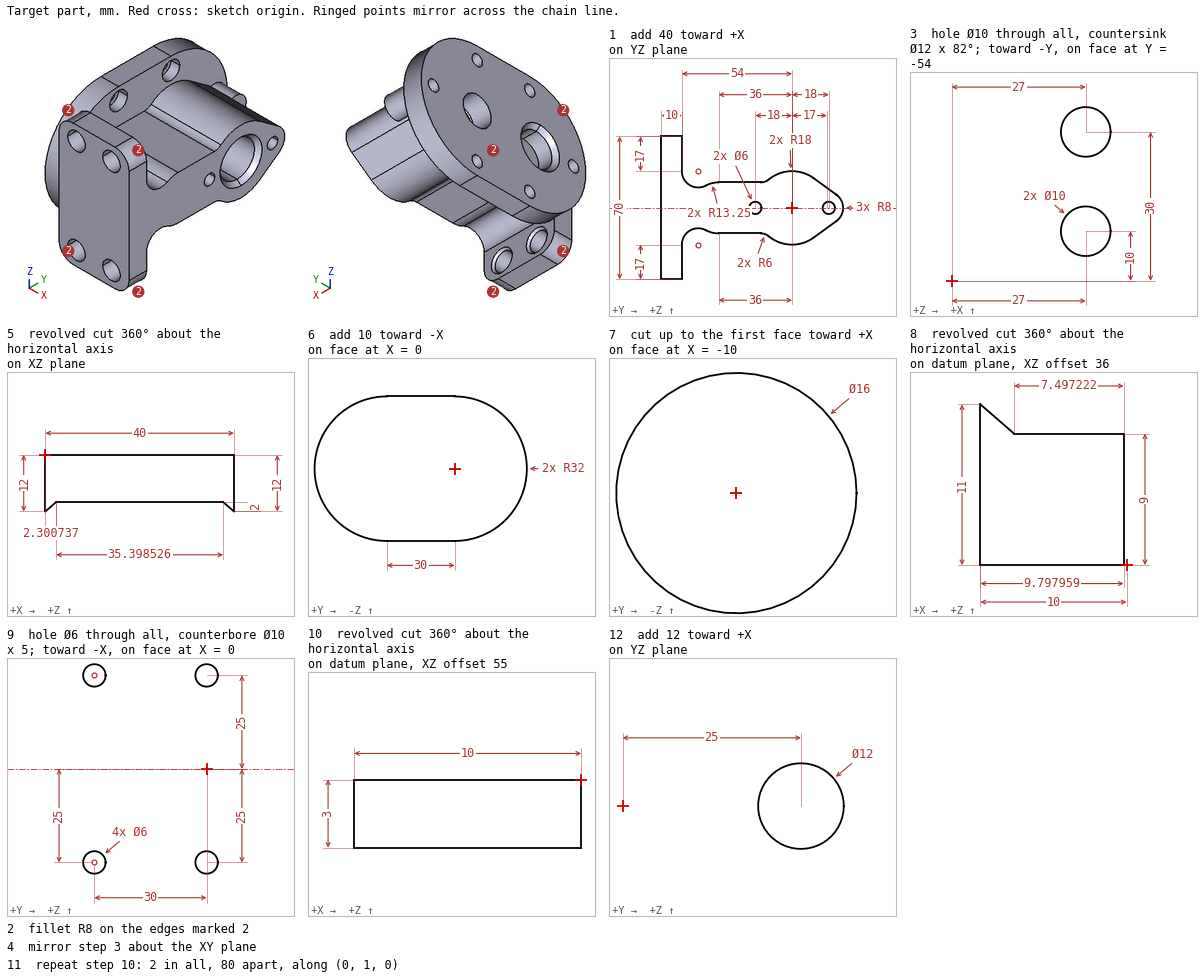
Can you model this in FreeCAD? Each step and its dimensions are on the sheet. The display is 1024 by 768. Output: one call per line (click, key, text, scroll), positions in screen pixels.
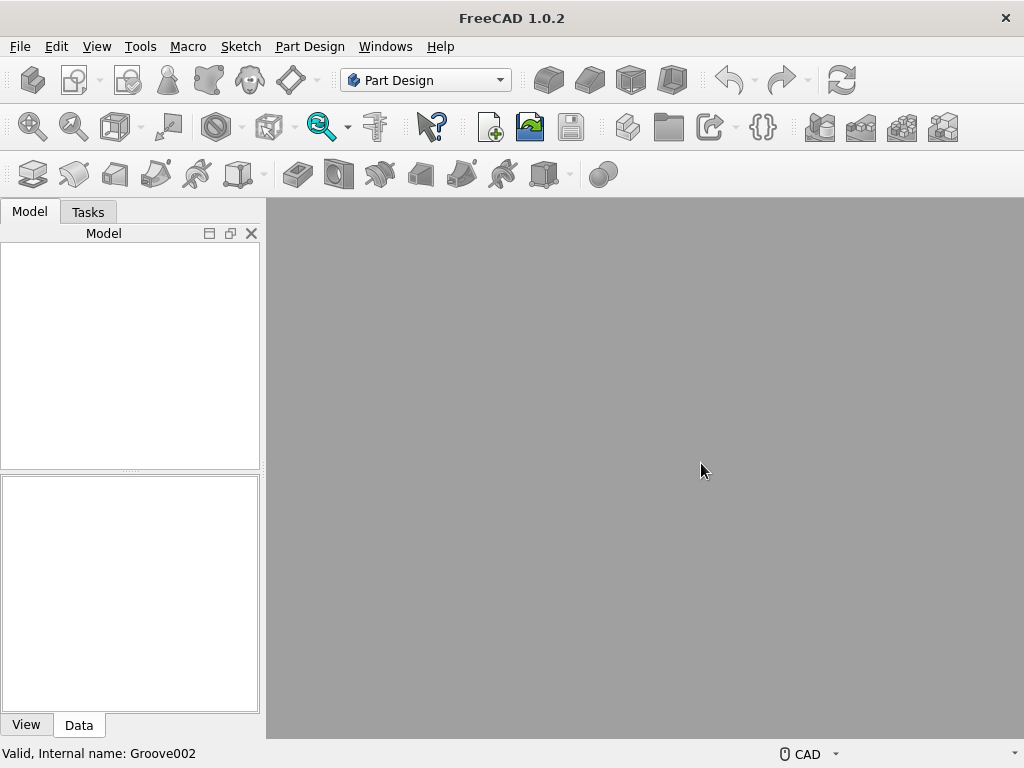
click(489, 128)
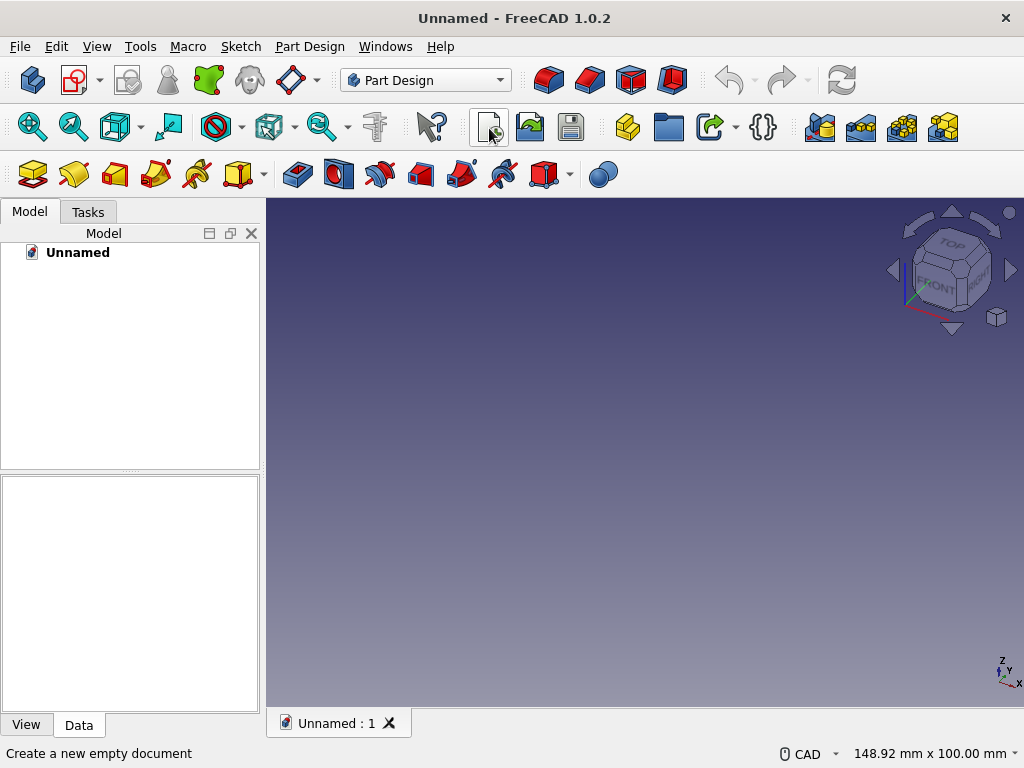
click(74, 80)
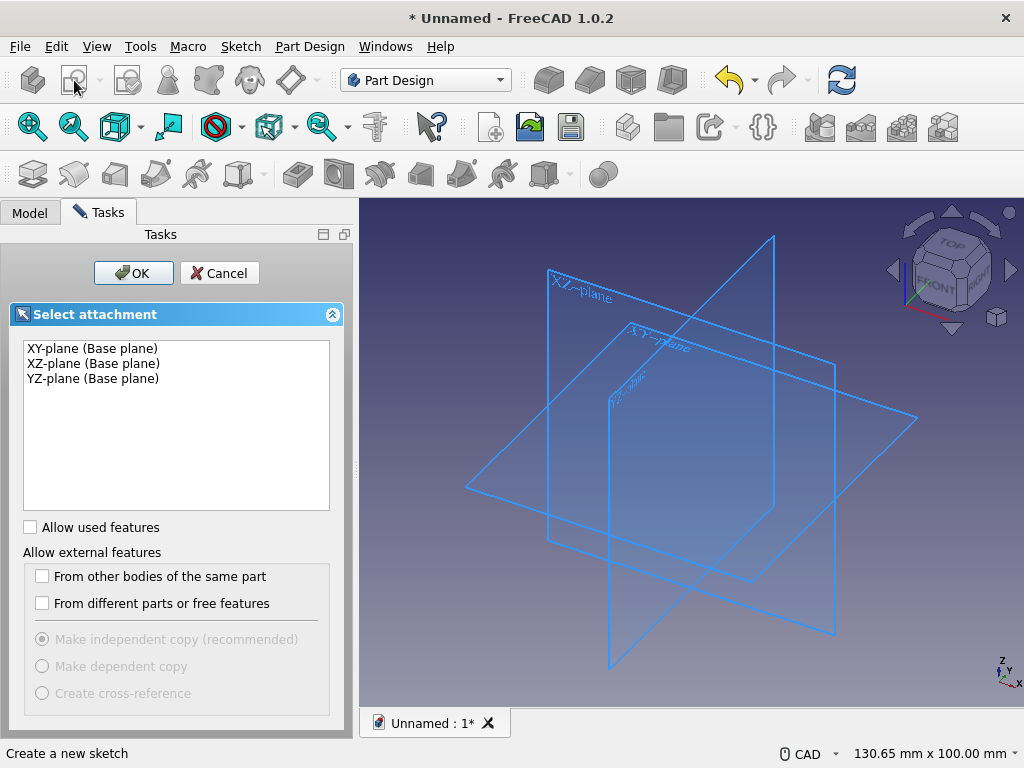
click(84, 378)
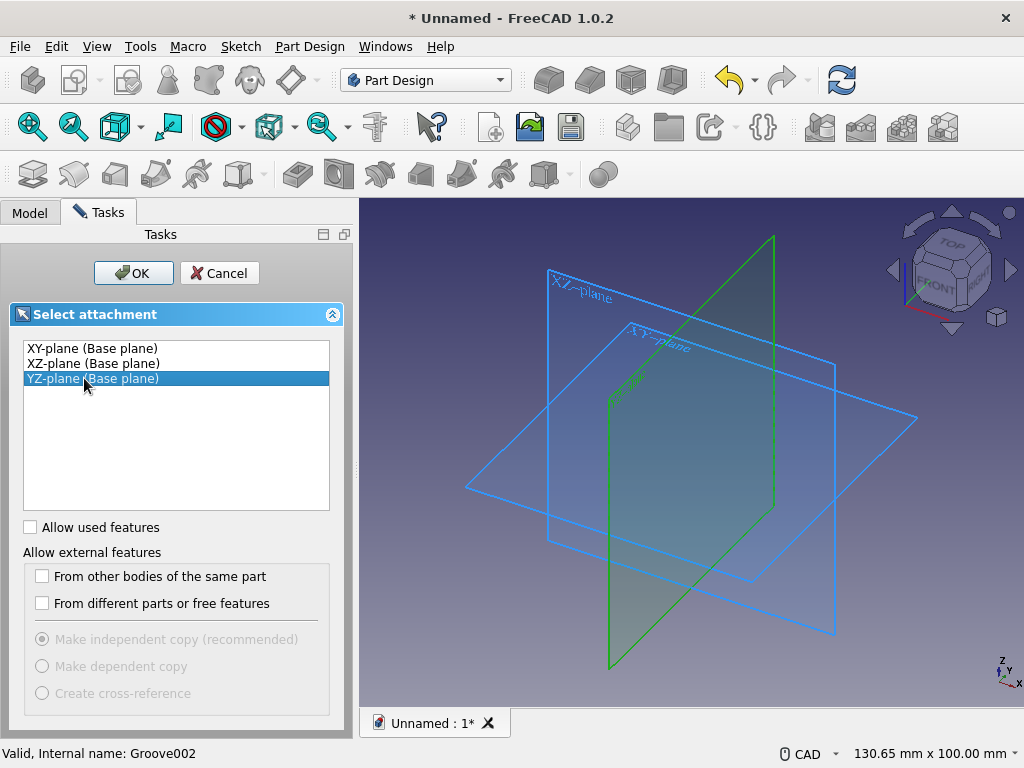
click(134, 273)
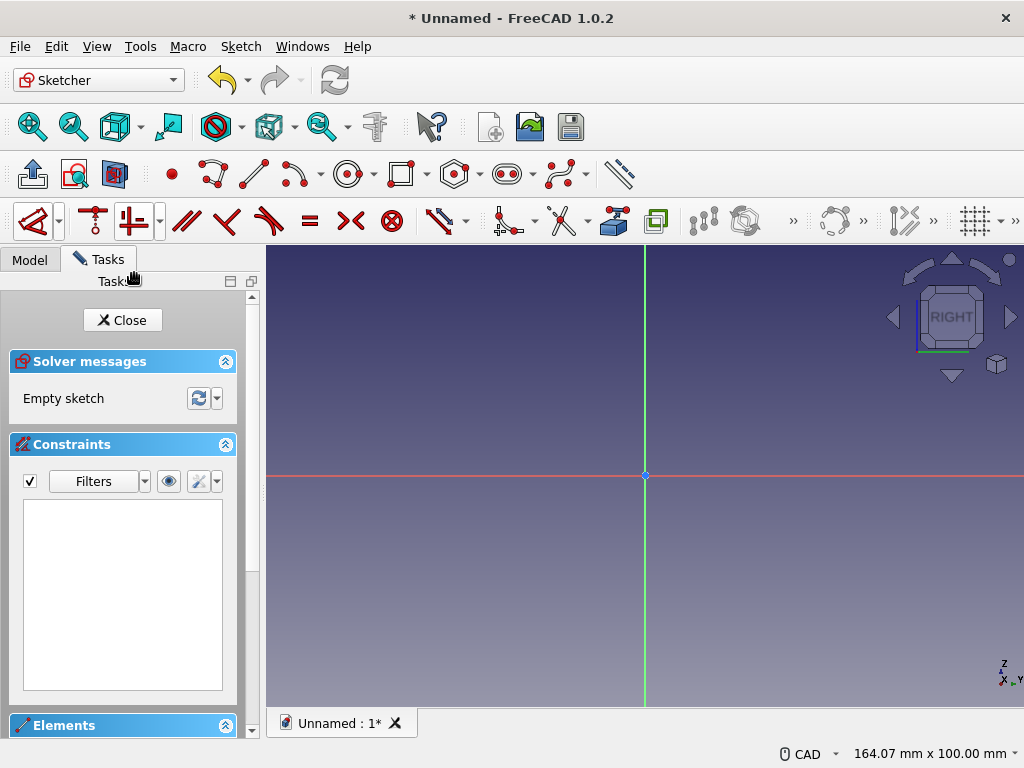
click(254, 174)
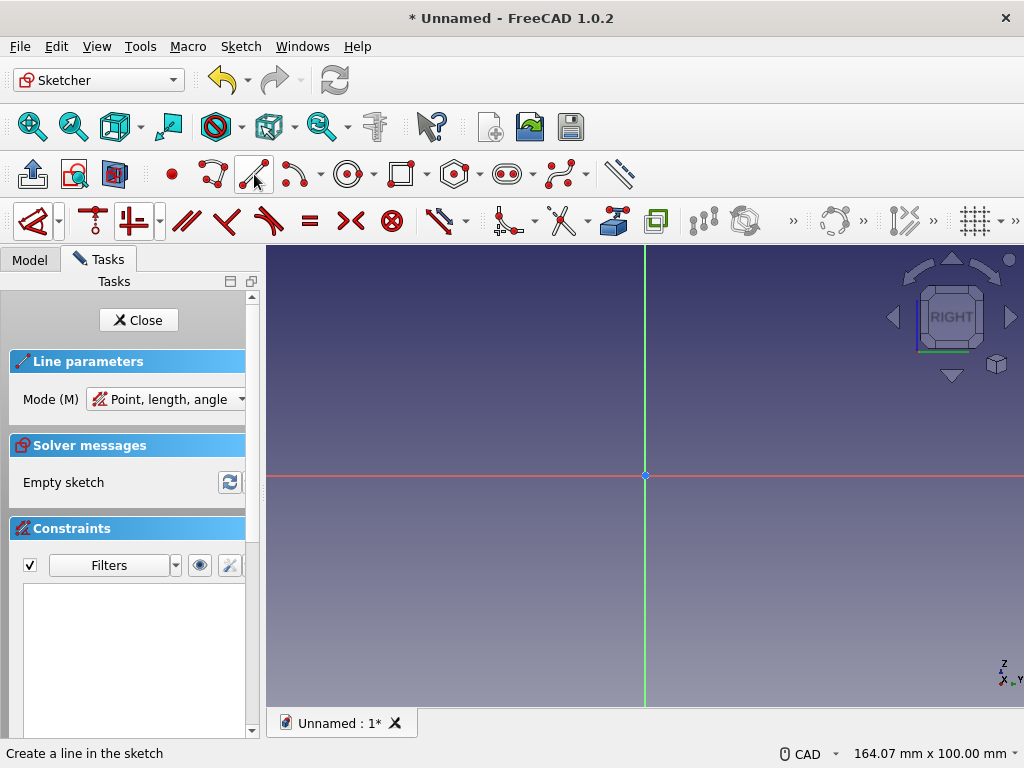
click(574, 418)
click(479, 418)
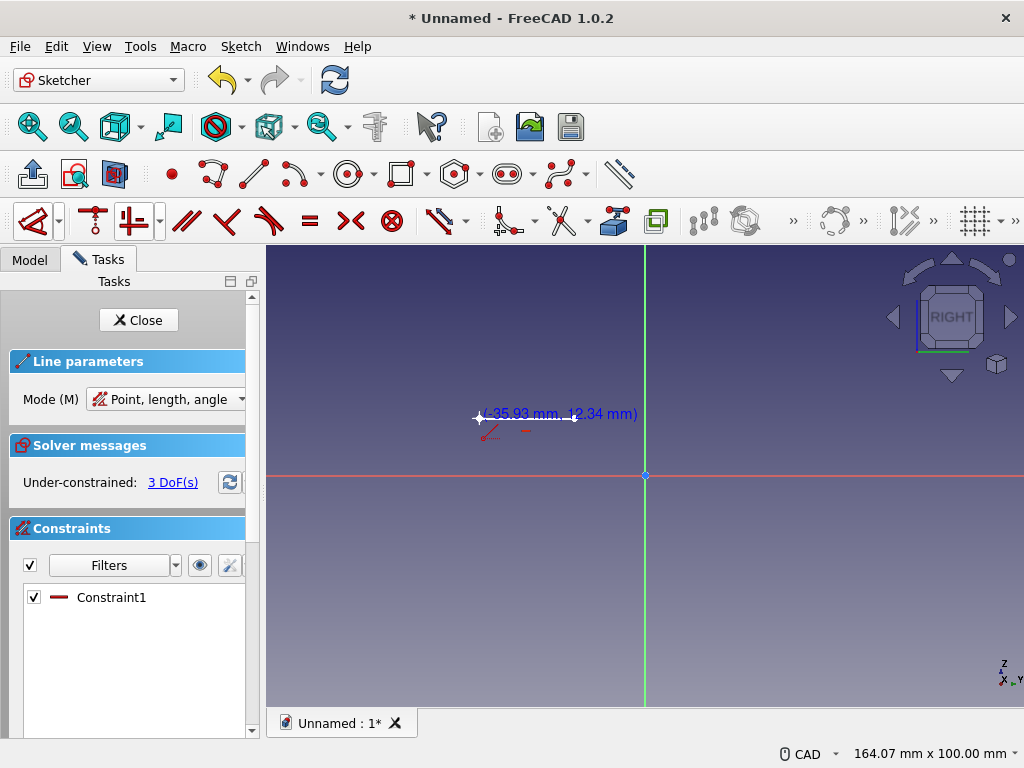
click(213, 174)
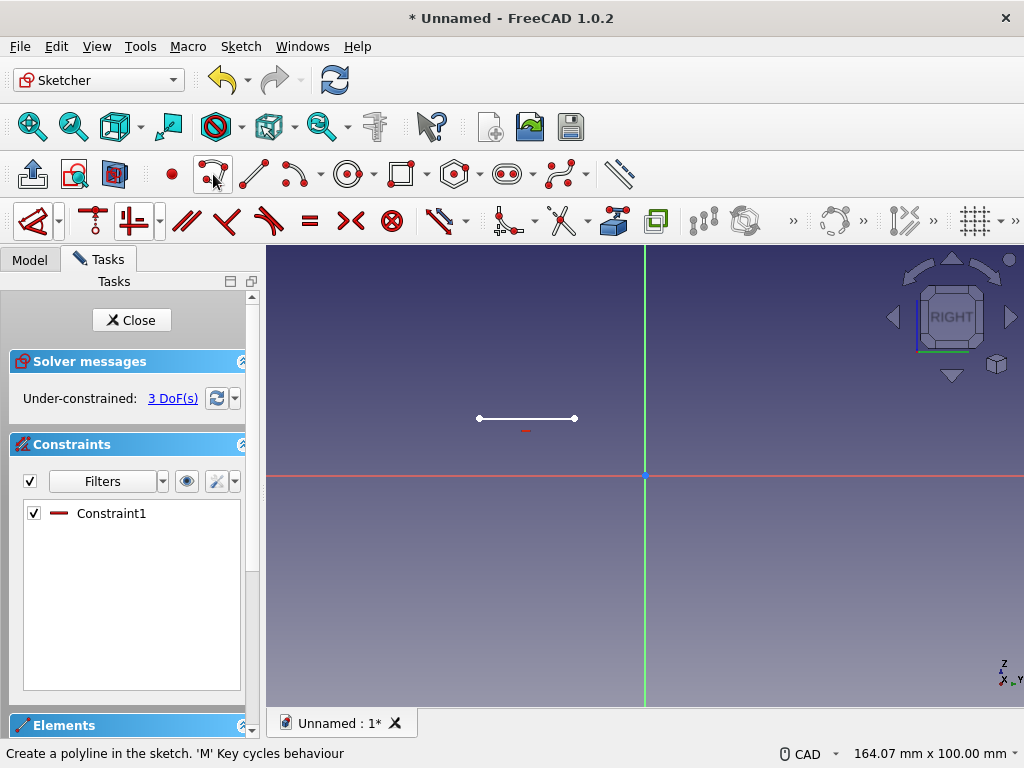
click(396, 393)
click(396, 314)
click(349, 314)
click(349, 638)
click(396, 638)
click(396, 559)
right_click(396, 559)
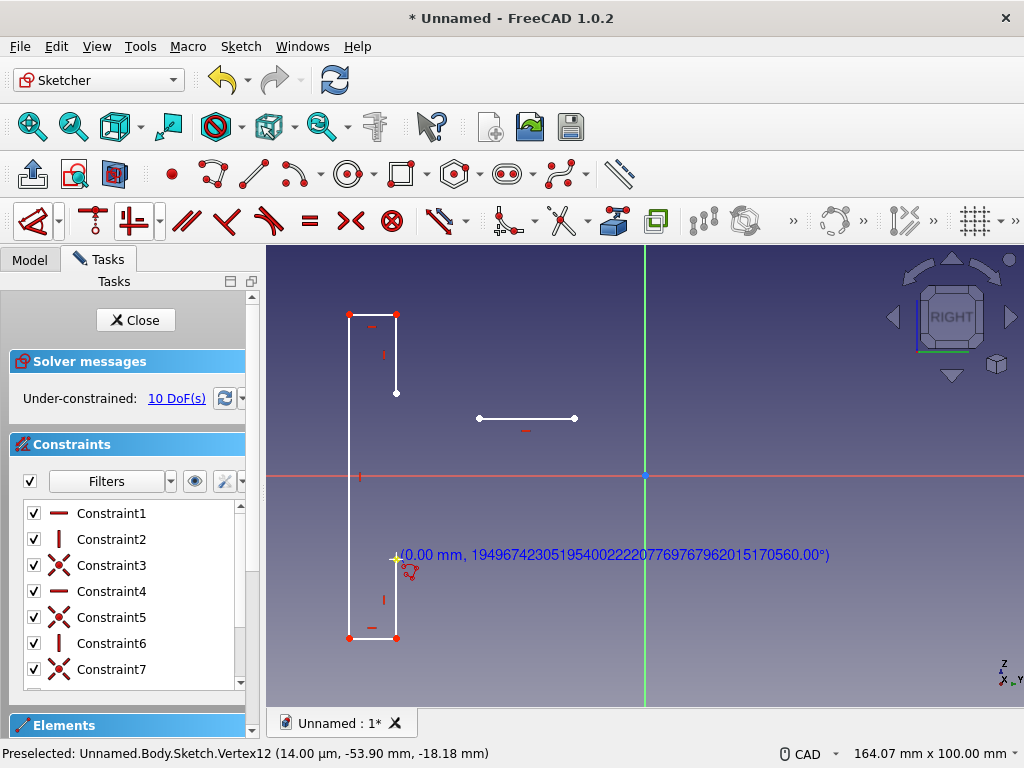
click(254, 174)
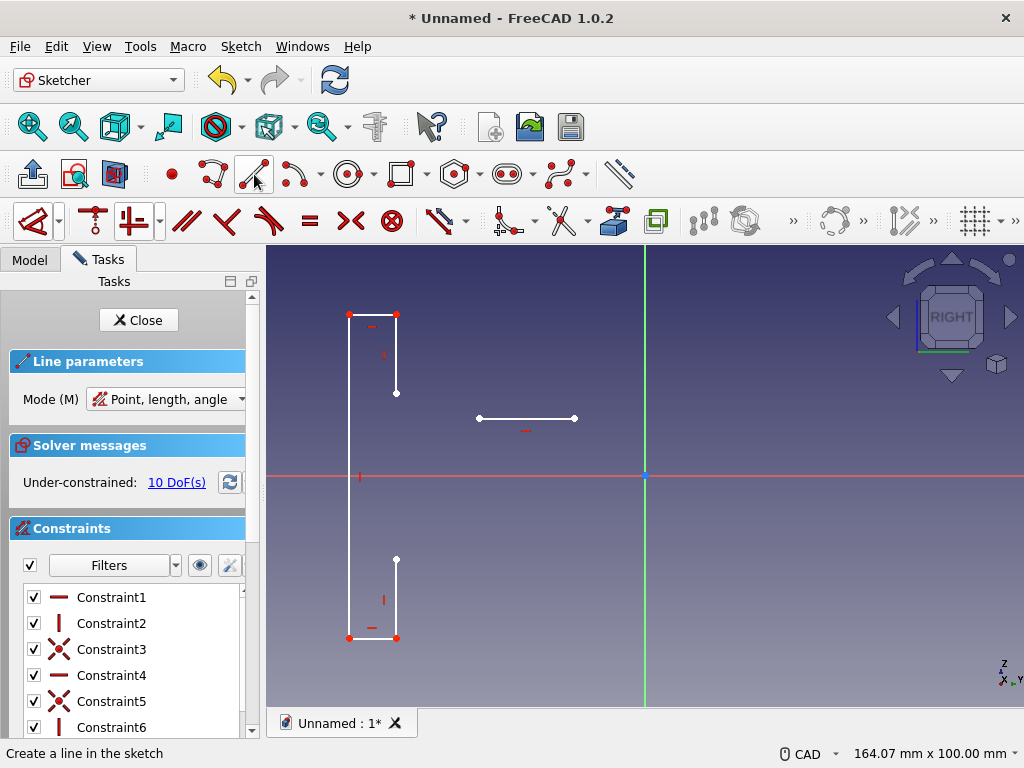
click(479, 534)
click(574, 534)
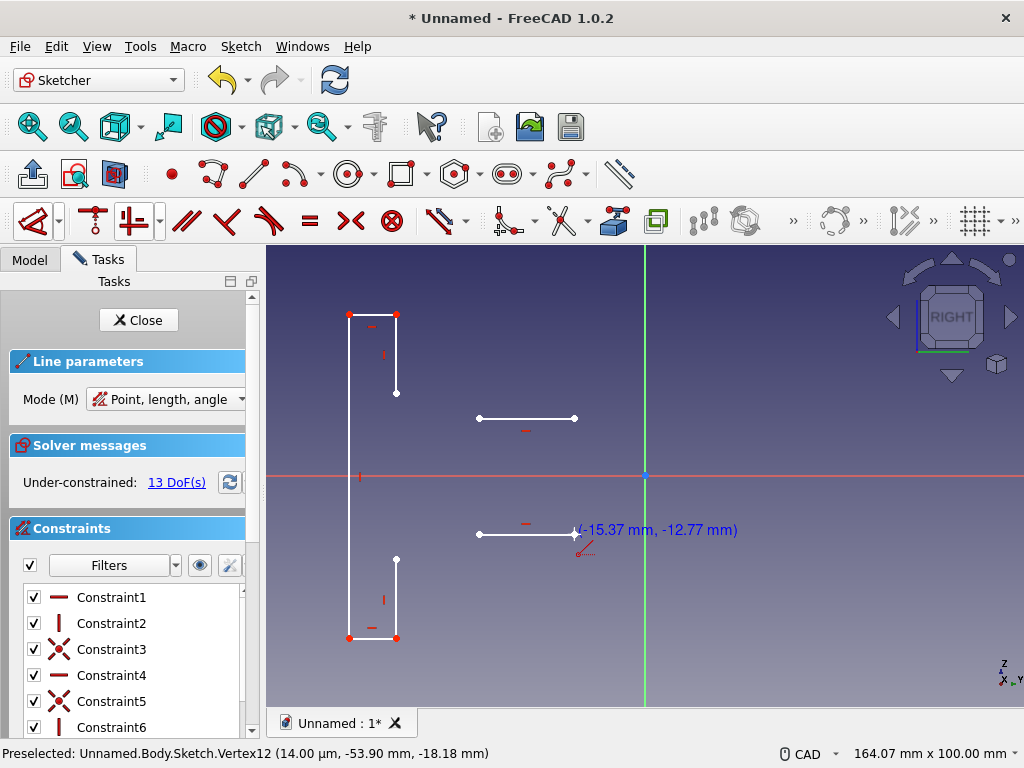
click(694, 543)
click(745, 506)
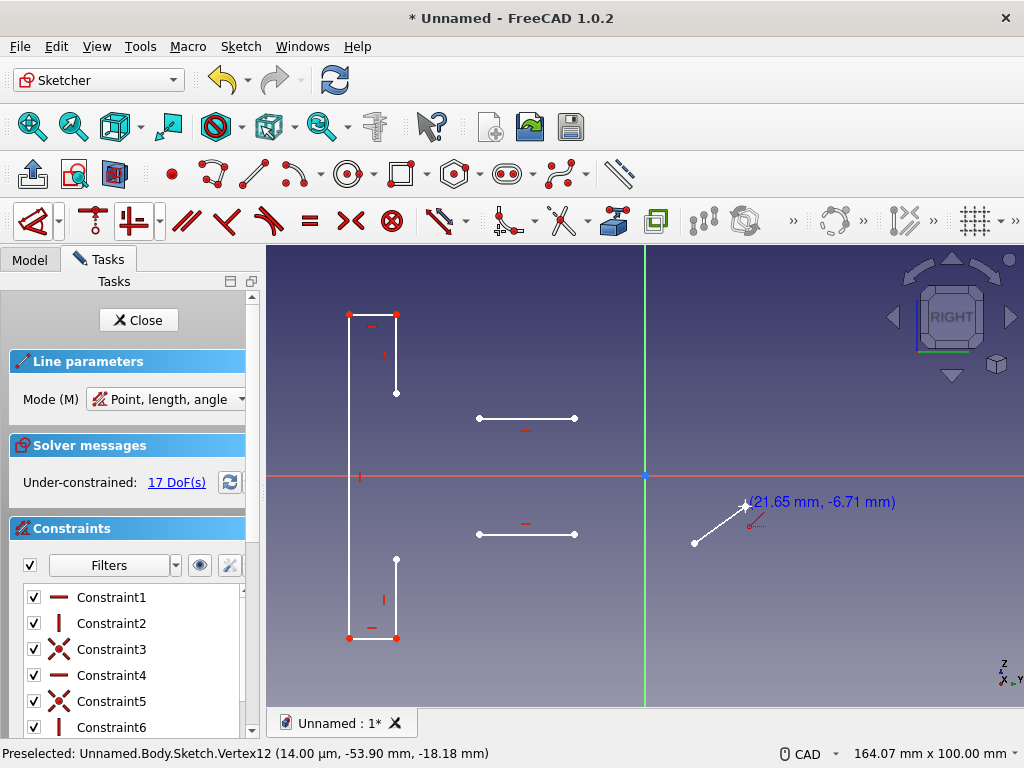
click(745, 446)
click(694, 409)